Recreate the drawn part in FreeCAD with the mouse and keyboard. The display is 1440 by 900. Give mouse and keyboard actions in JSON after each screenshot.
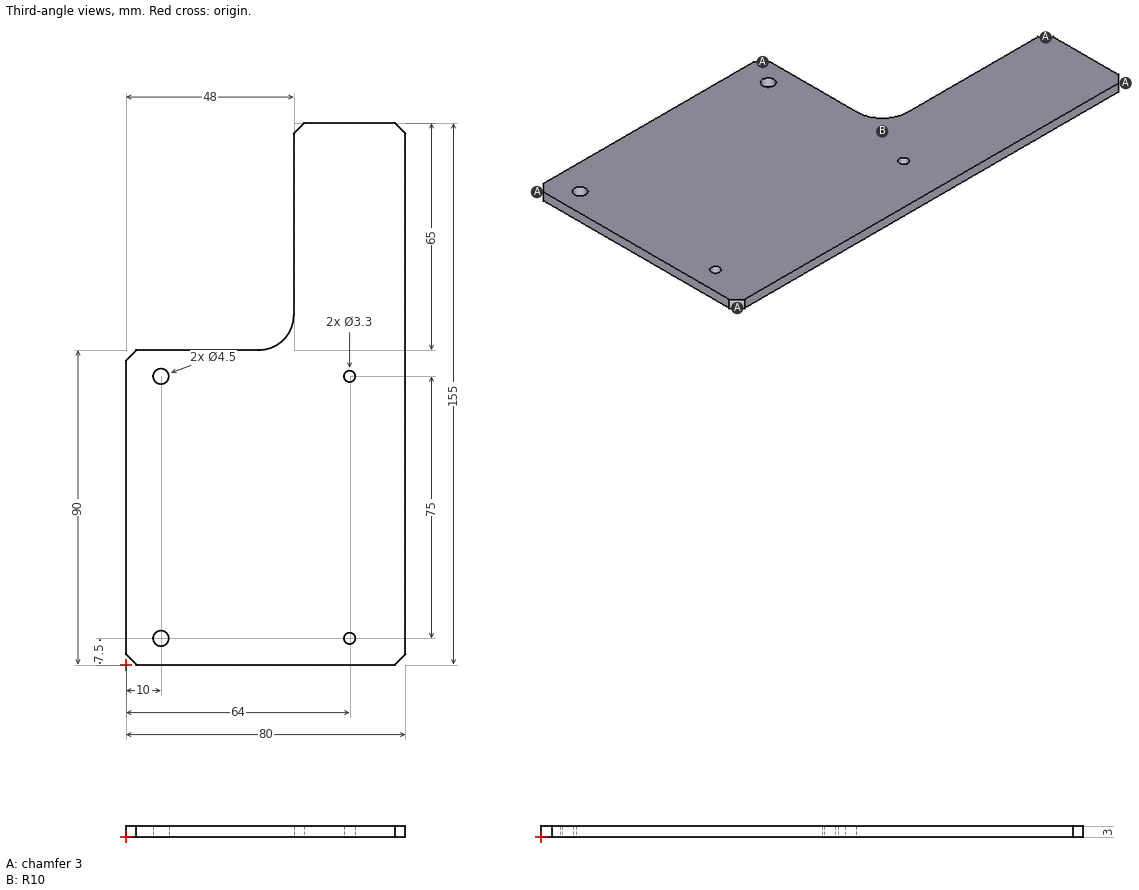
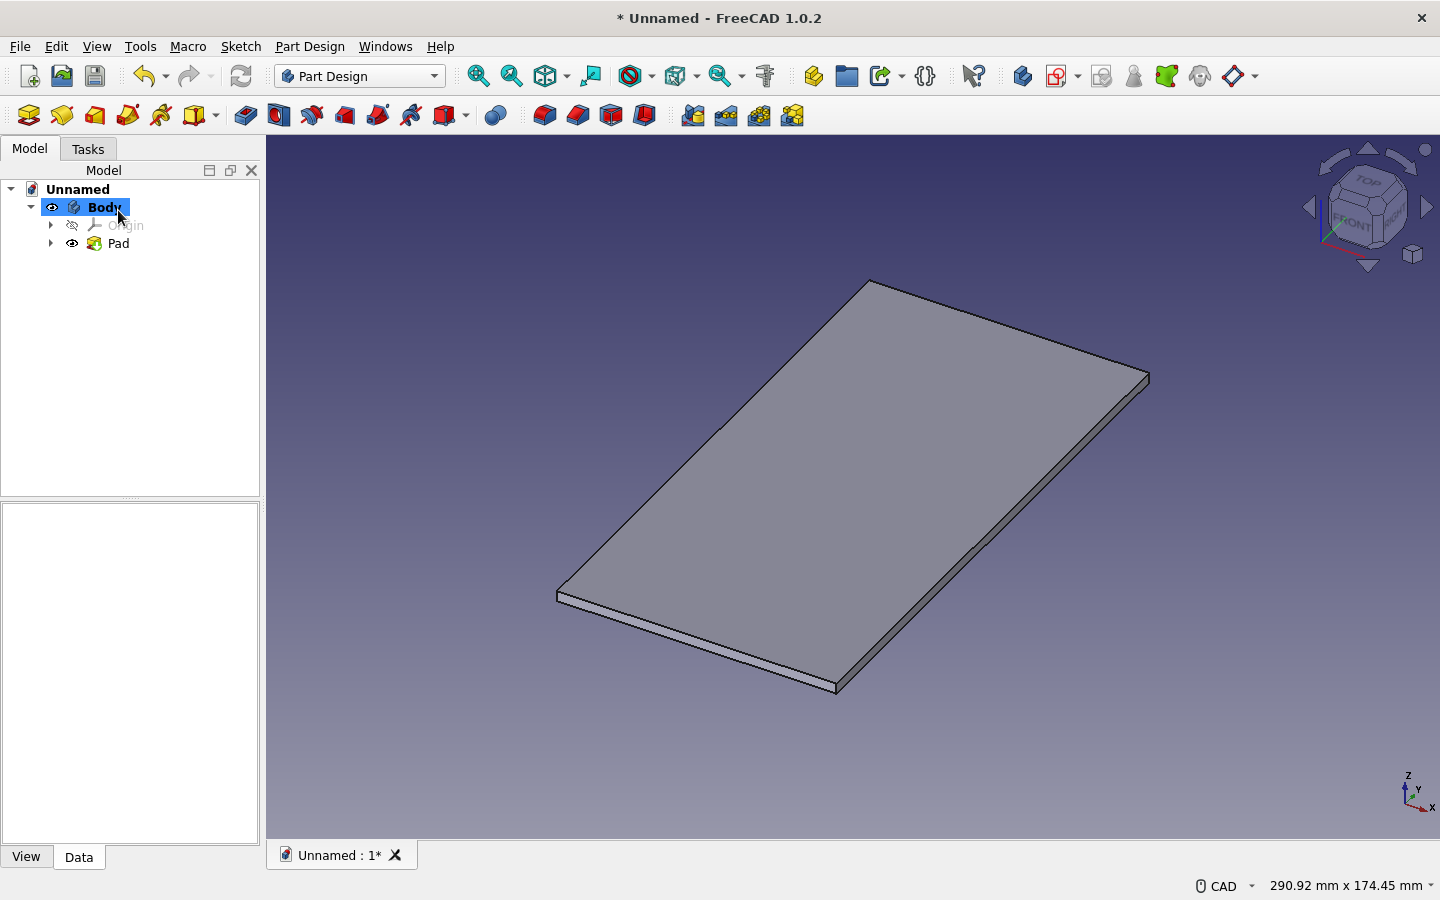
{"action": "left_click", "coordinate": [898, 437]}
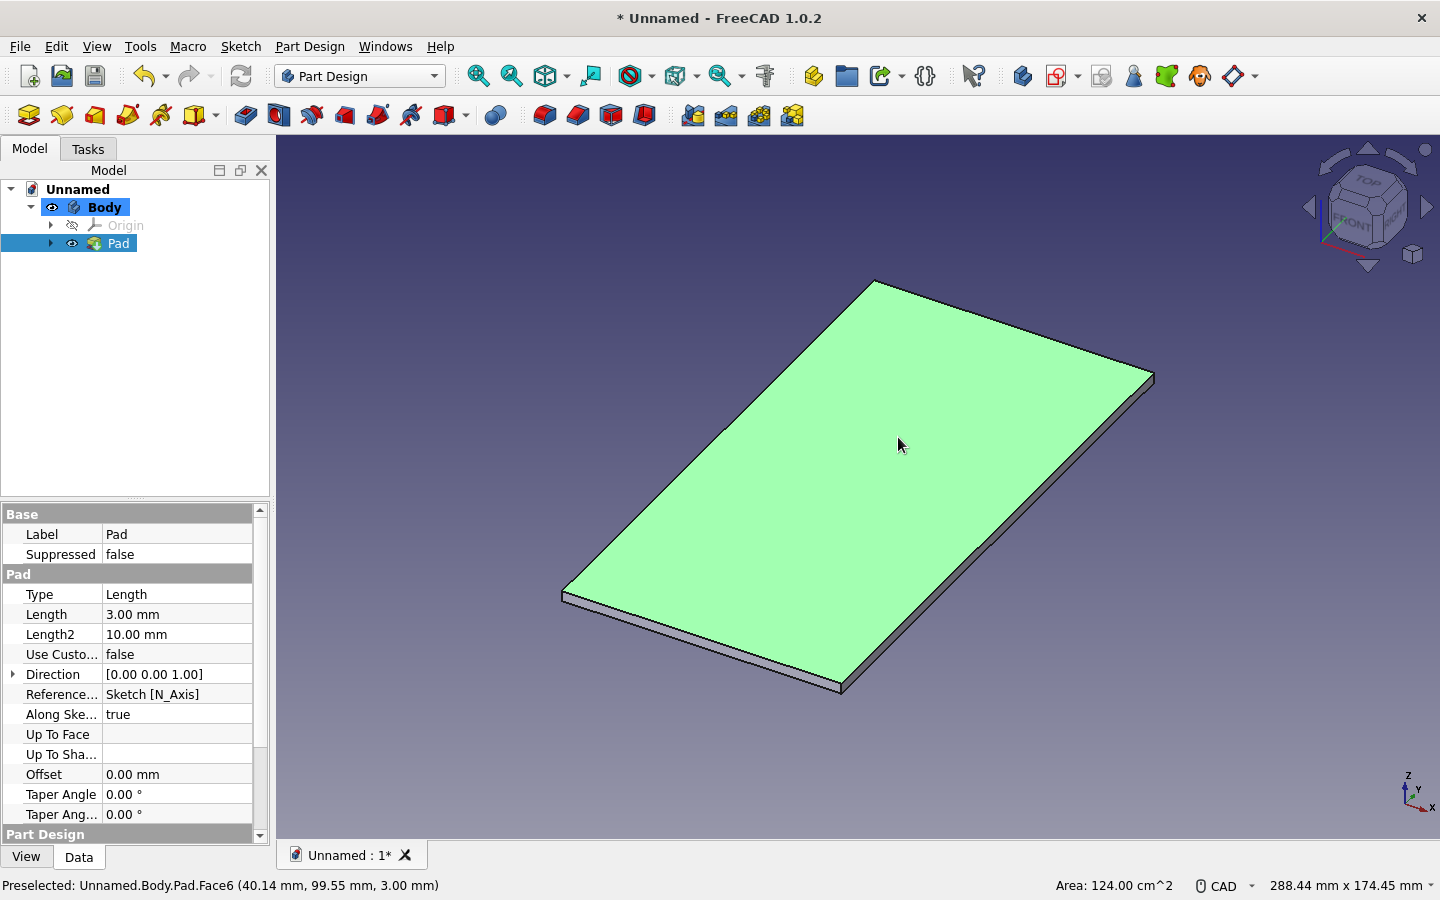
{"action": "left_click", "coordinate": [1056, 76]}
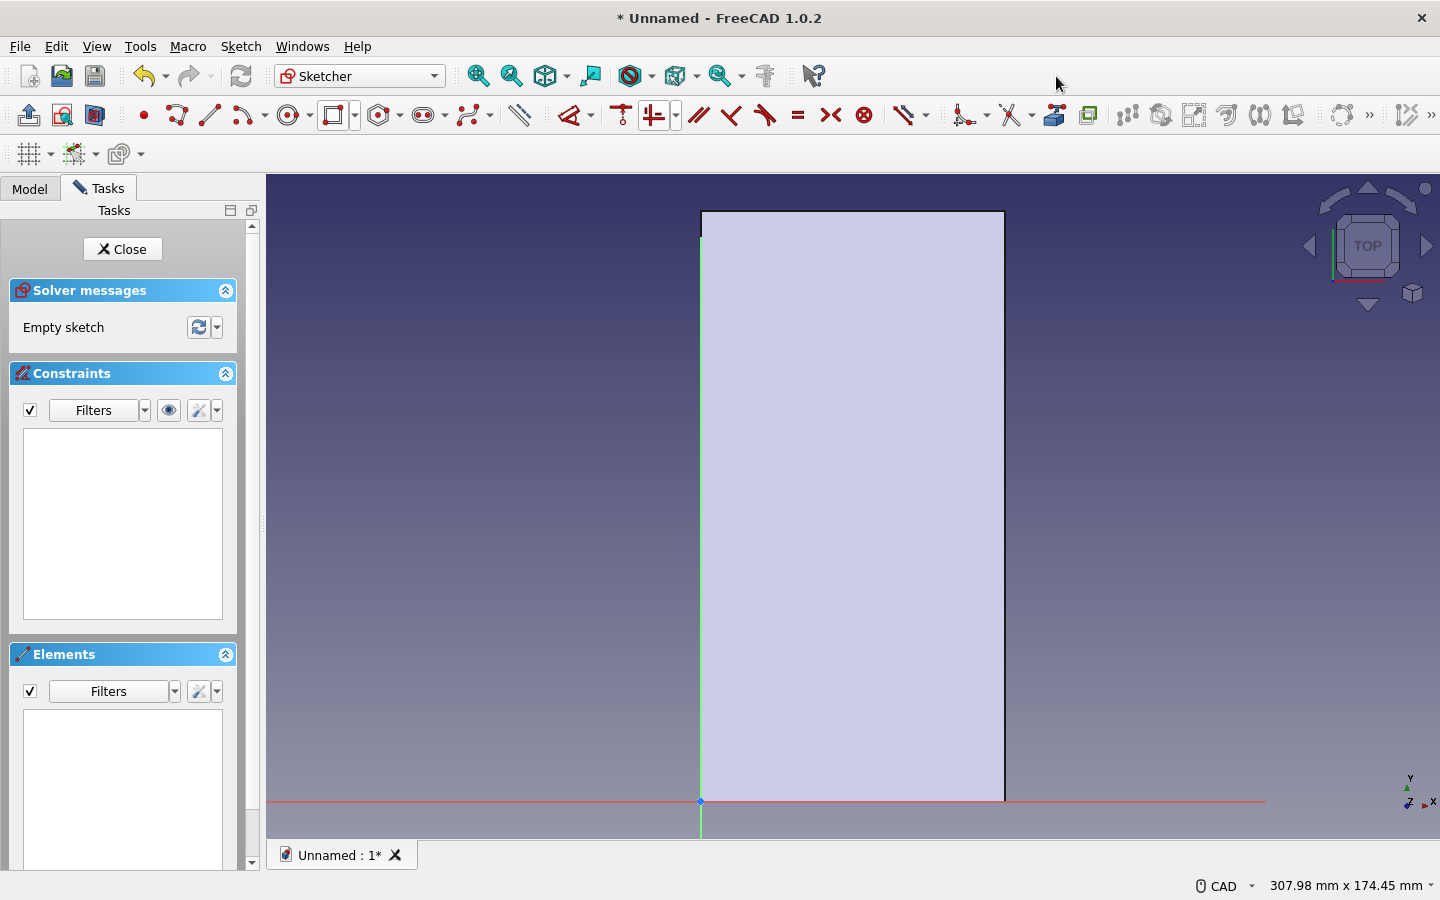
{"action": "scroll", "coordinate": [599, 202], "scroll_direction": "down", "scroll_amount": 1}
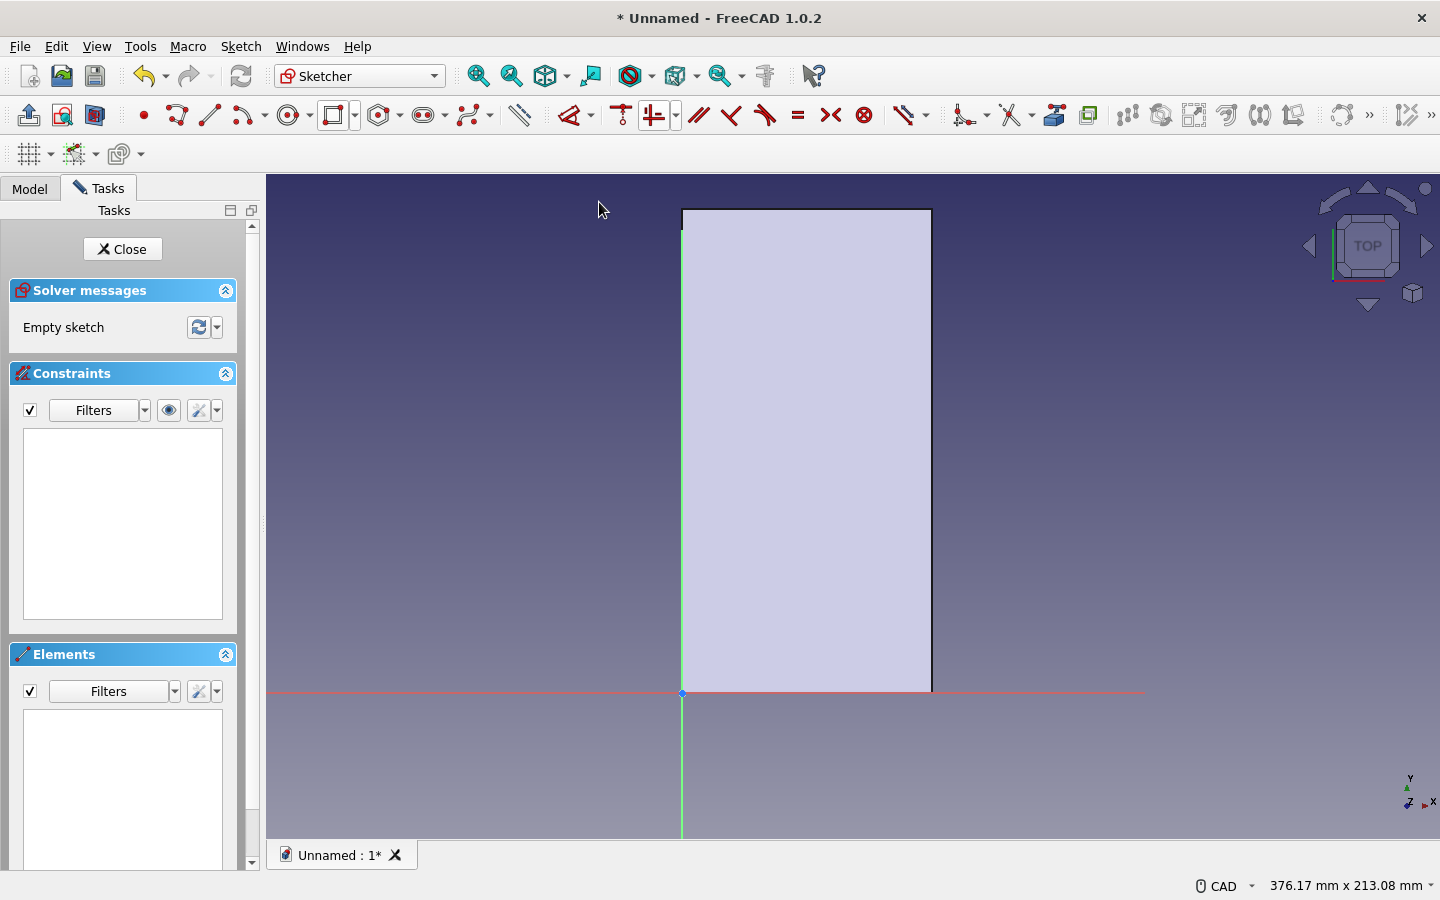
{"action": "scroll", "coordinate": [785, 674], "scroll_direction": "up", "scroll_amount": 2}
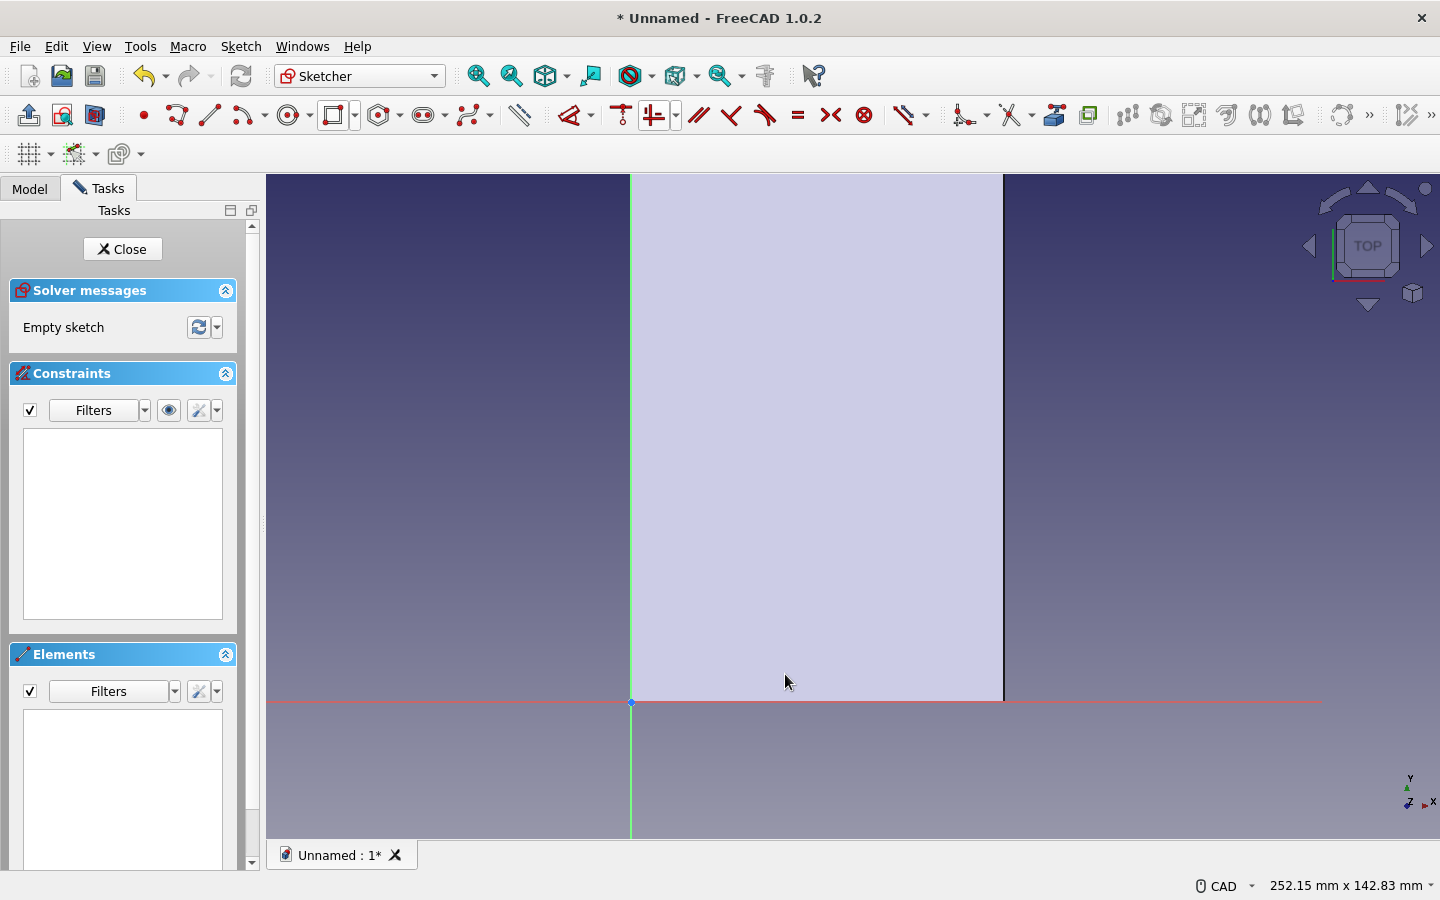
{"action": "key", "text": "g c"}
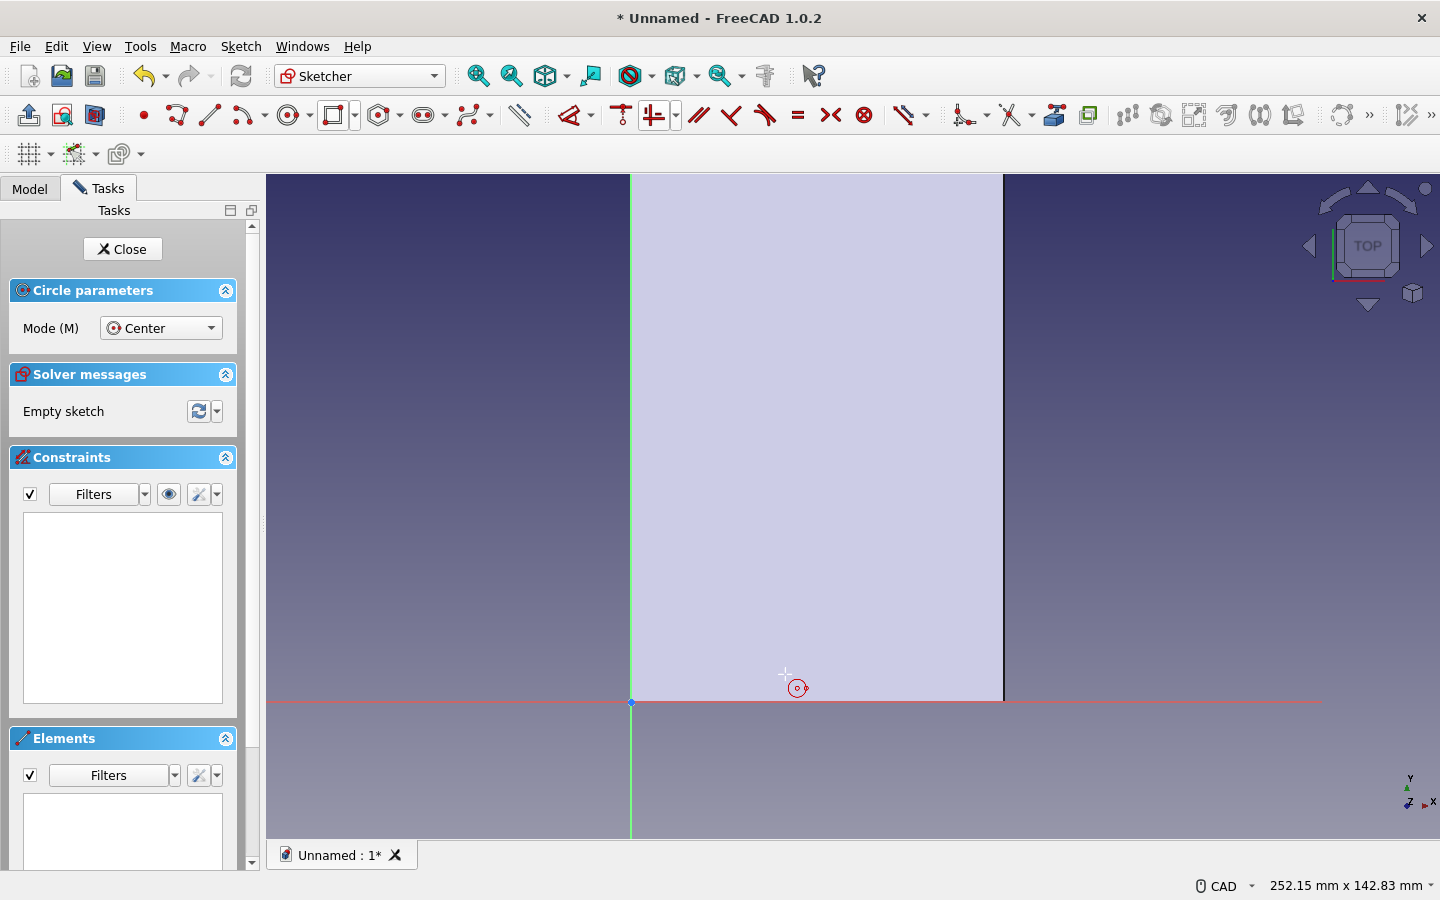
{"action": "scroll", "coordinate": [929, 318], "scroll_direction": "up", "scroll_amount": 6}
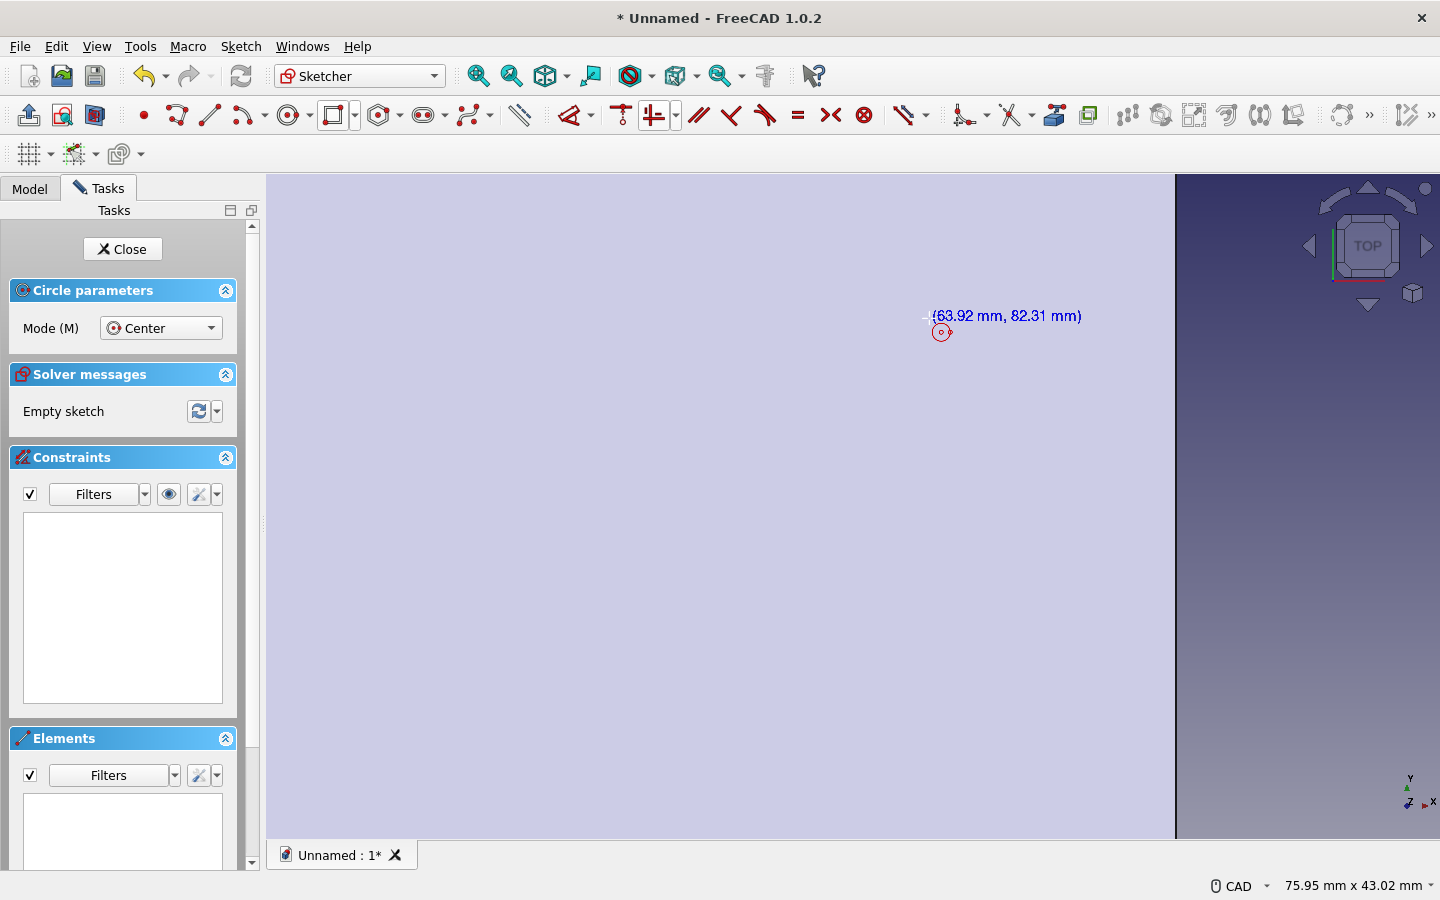
{"action": "left_click", "coordinate": [929, 318]}
{"action": "mouse_move", "coordinate": [947, 300]}